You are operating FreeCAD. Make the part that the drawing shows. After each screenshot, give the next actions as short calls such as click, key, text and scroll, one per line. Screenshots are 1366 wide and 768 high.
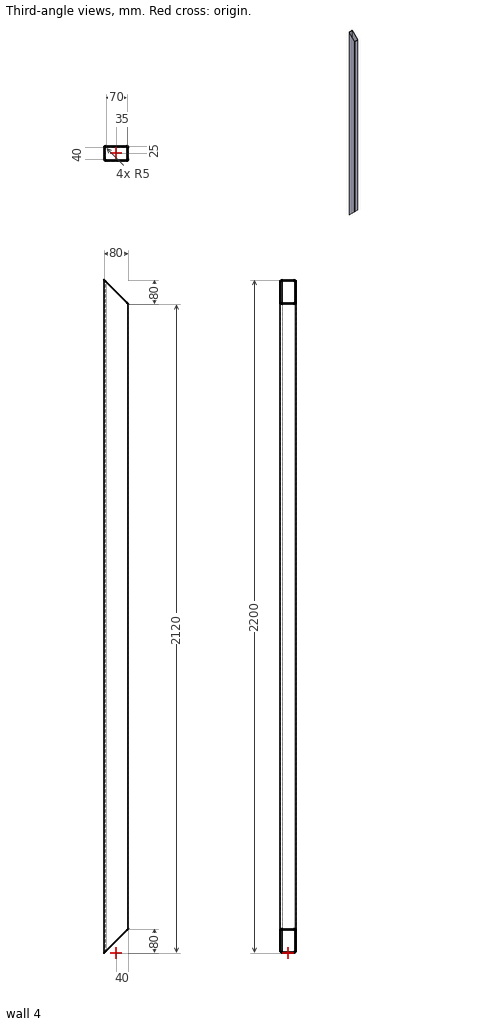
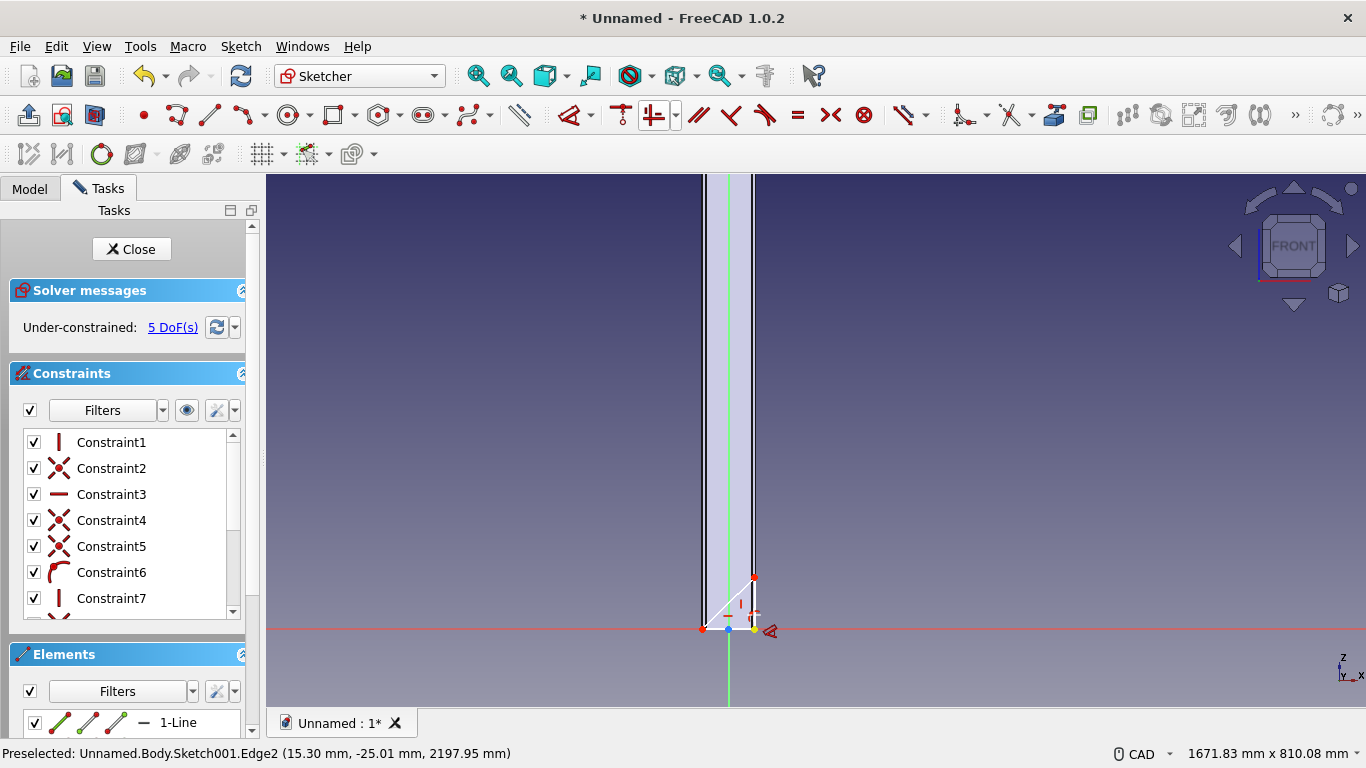
click(755, 614)
click(789, 603)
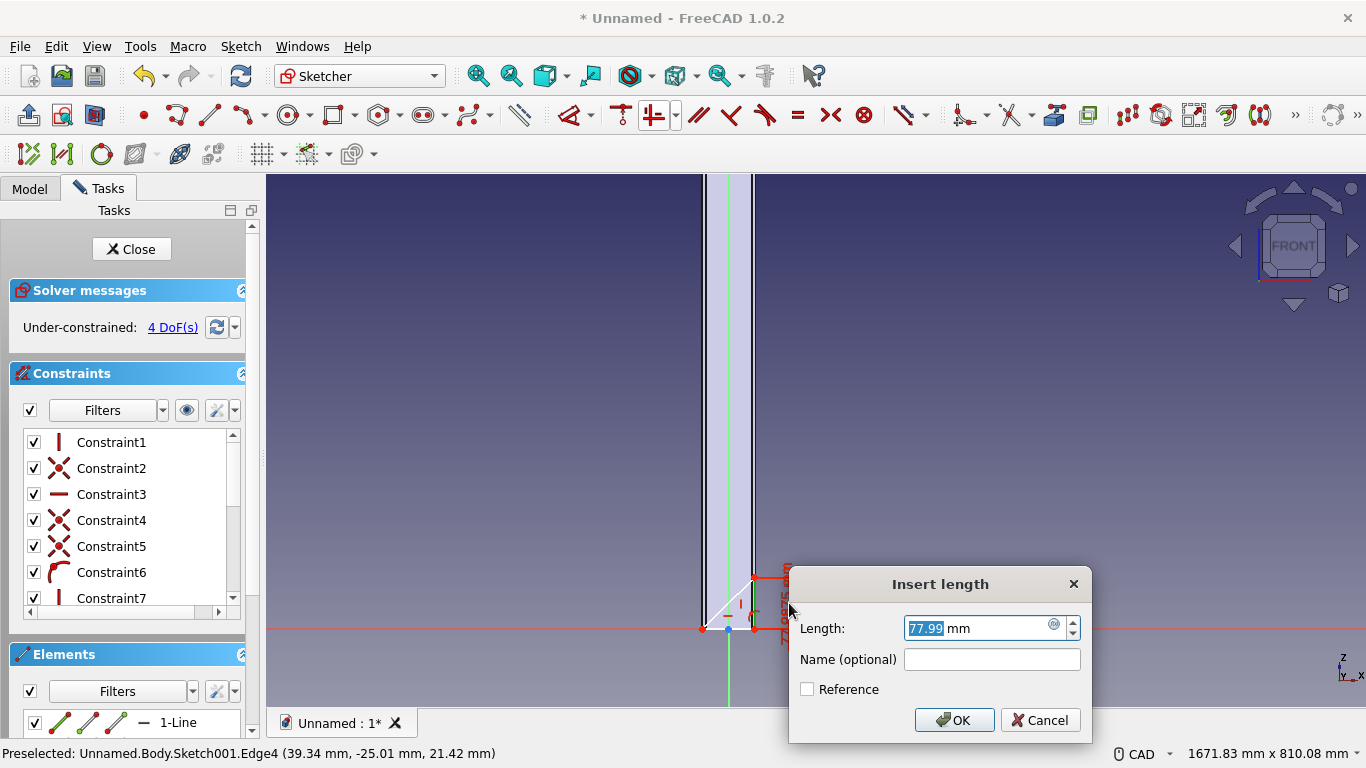
text(80)
key(Return)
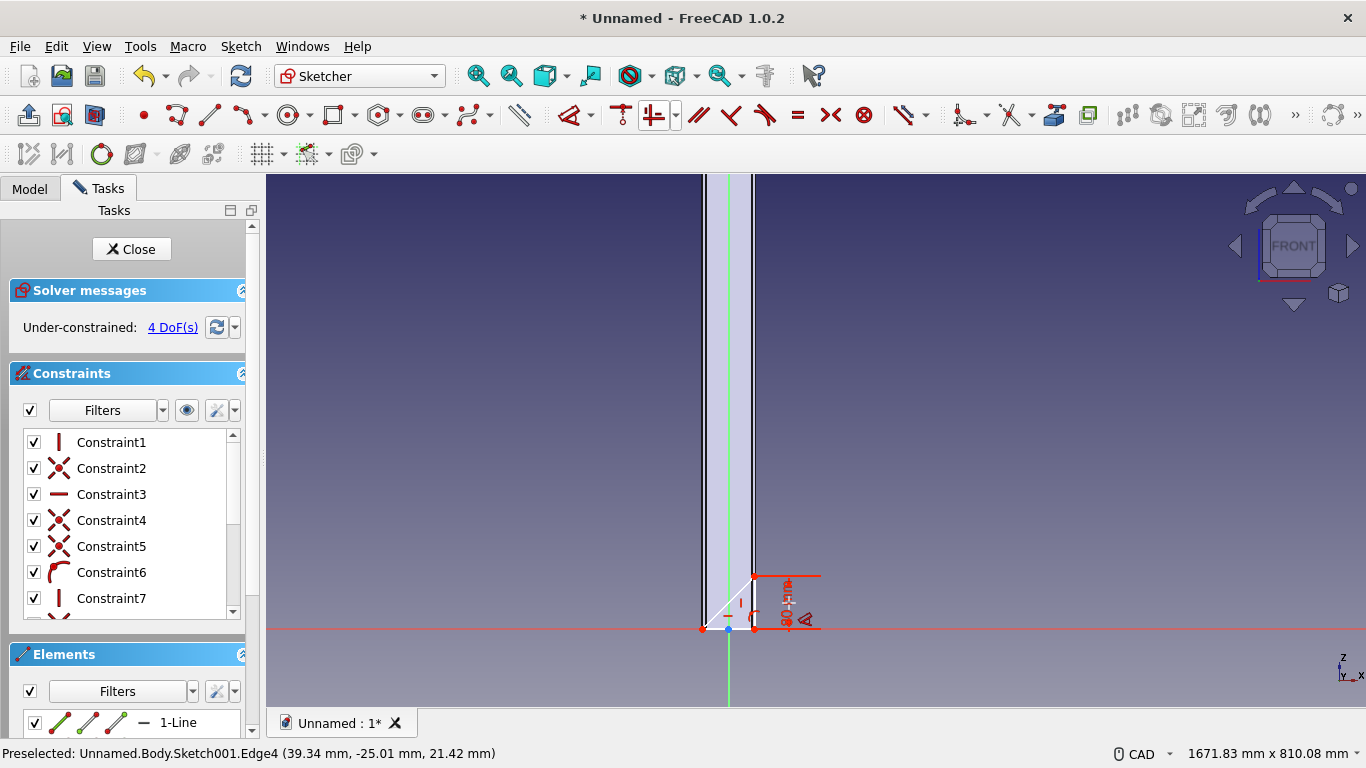
scroll(718, 629, up, 2)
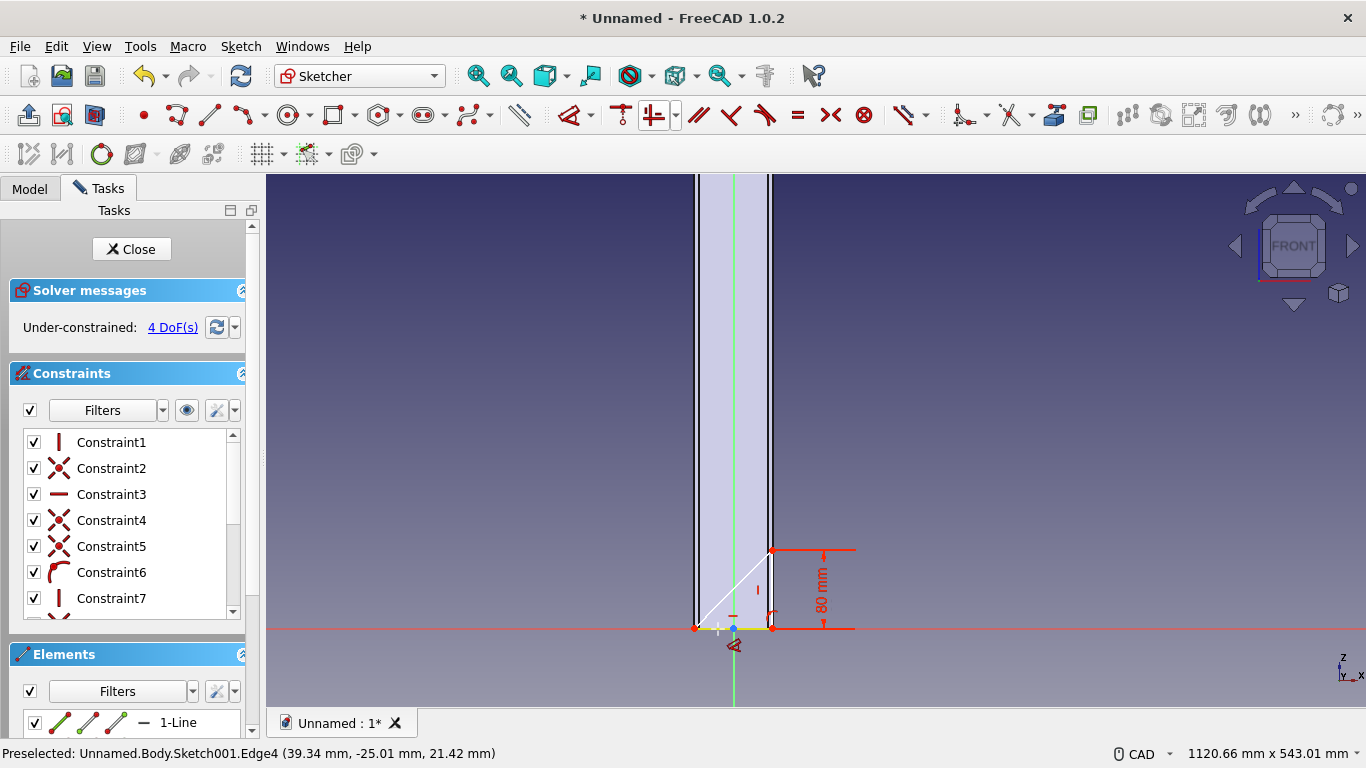
click(718, 629)
click(715, 663)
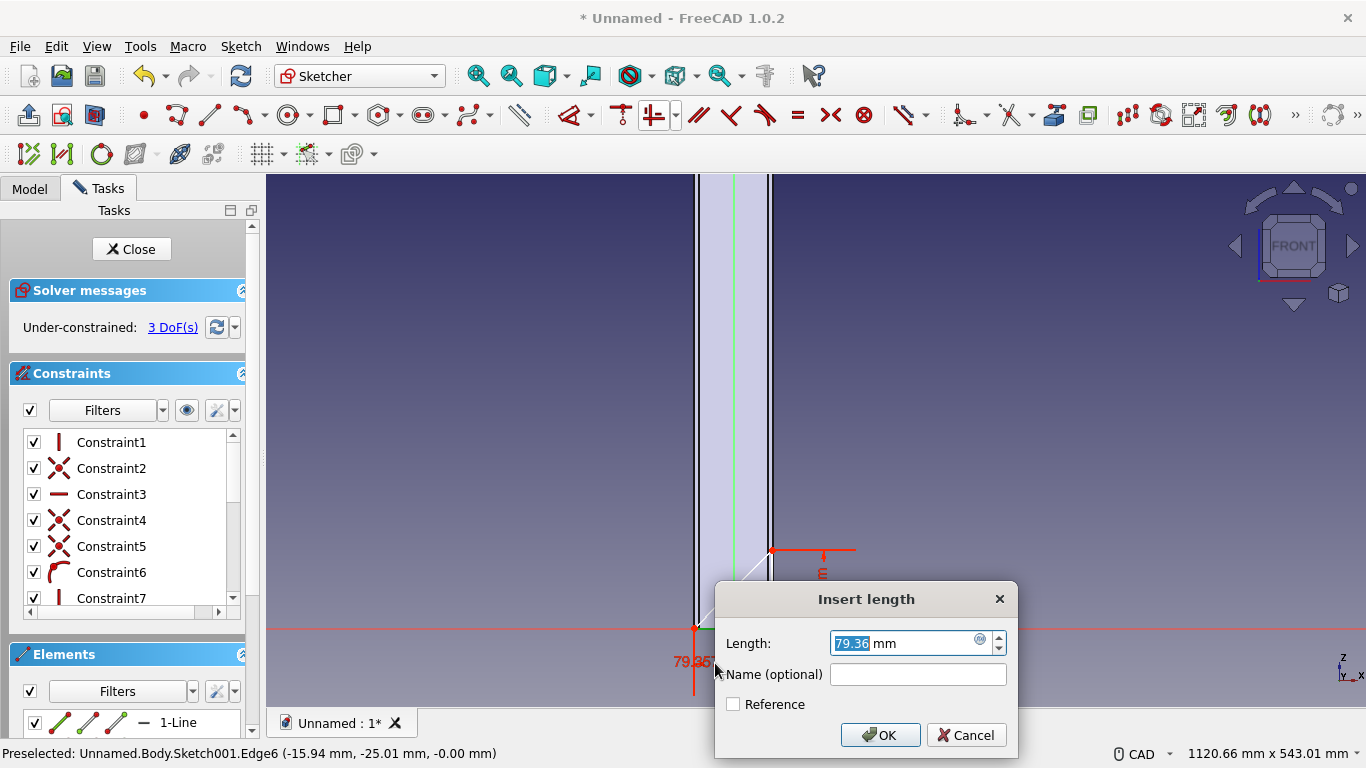
text(80)
key(Return)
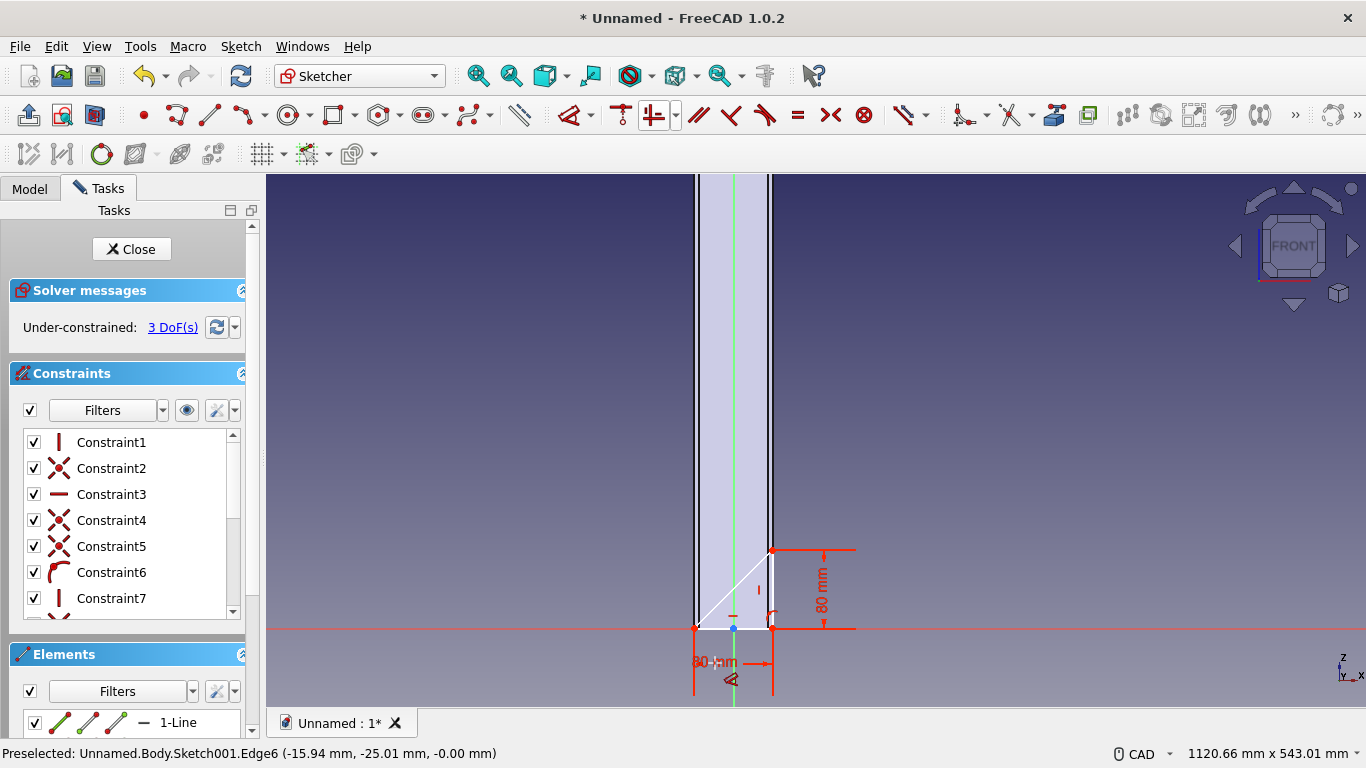
scroll(750, 617, down, 9)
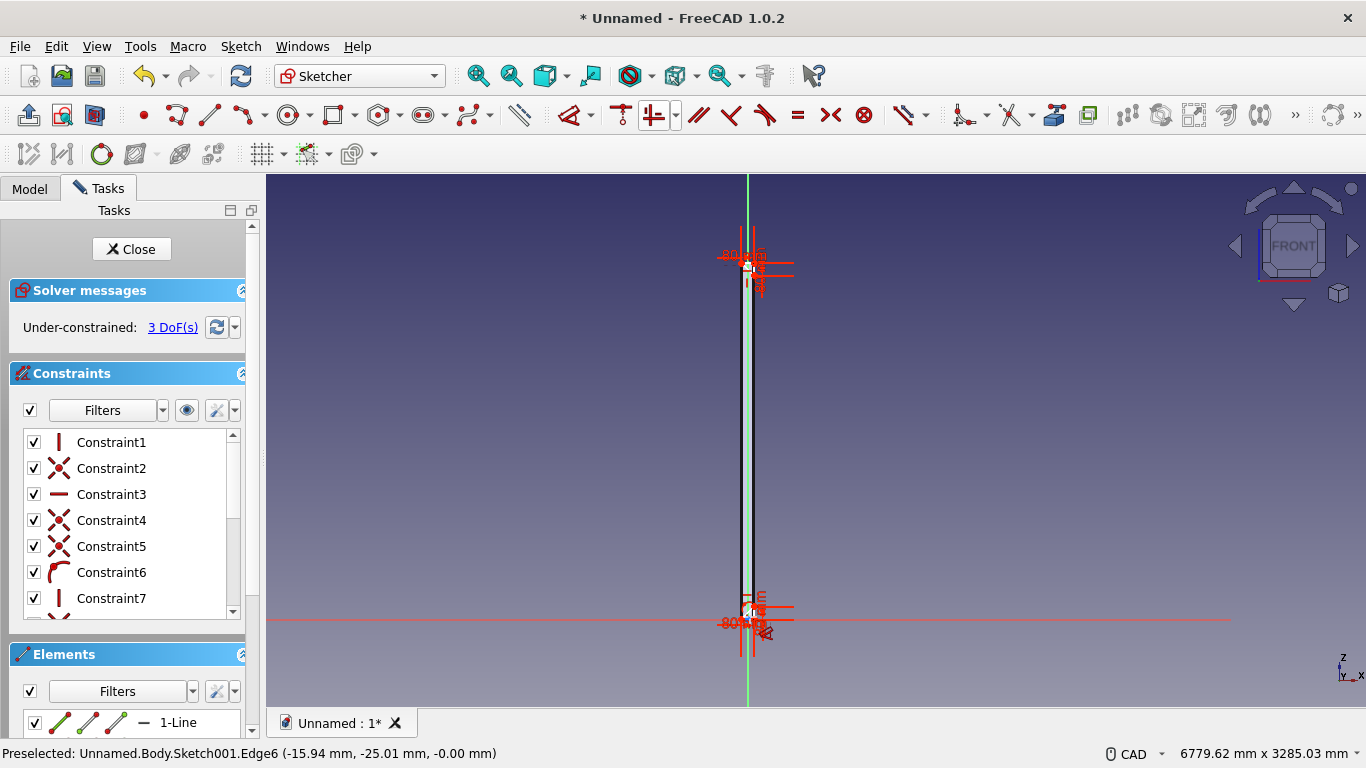
scroll(754, 276, up, 10)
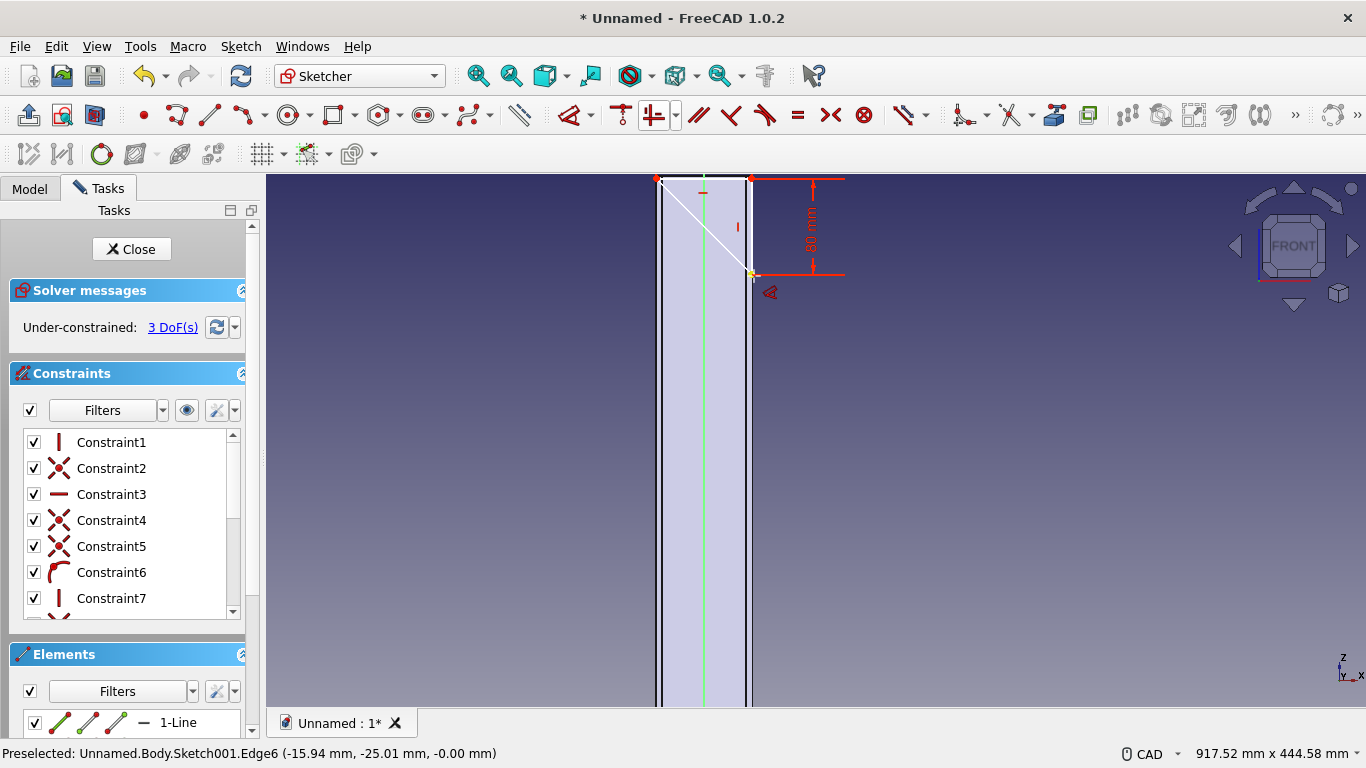
click(752, 275)
click(728, 217)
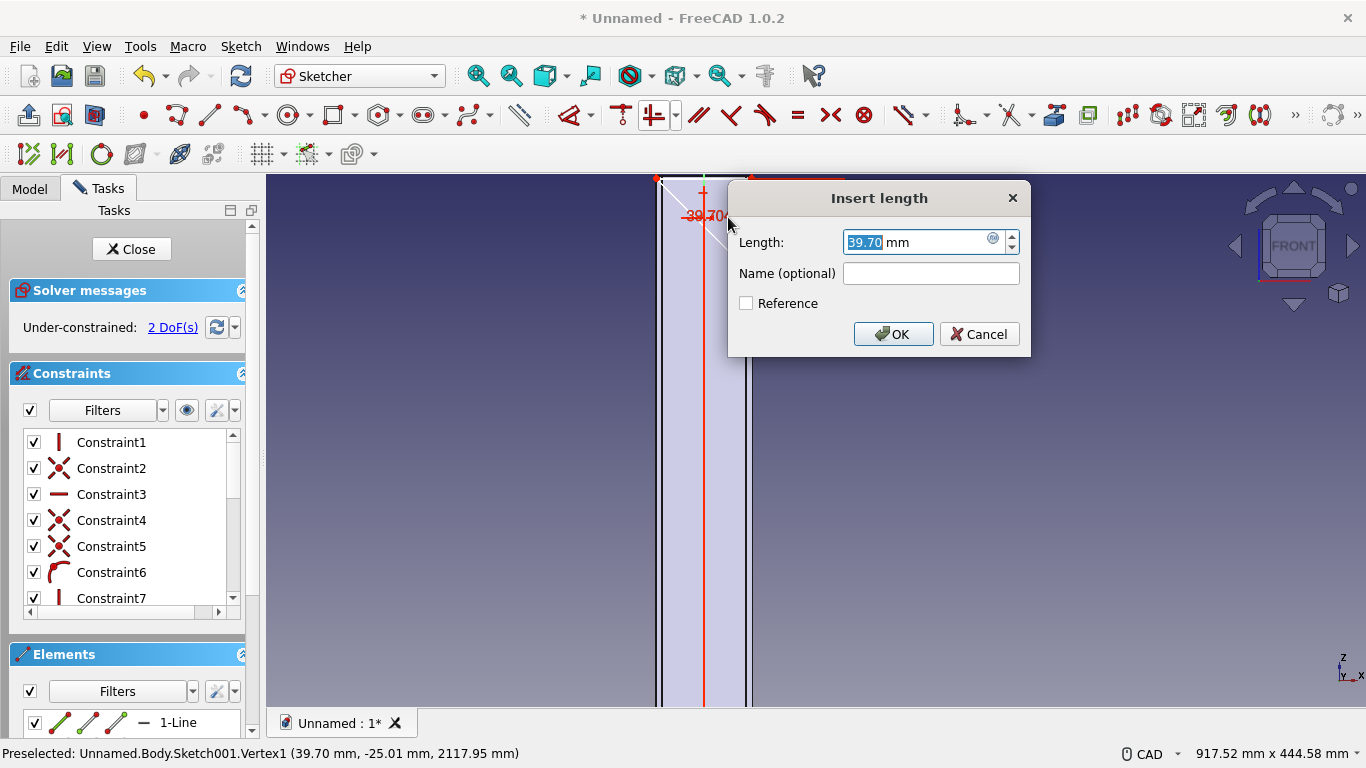
text(40)
key(Return)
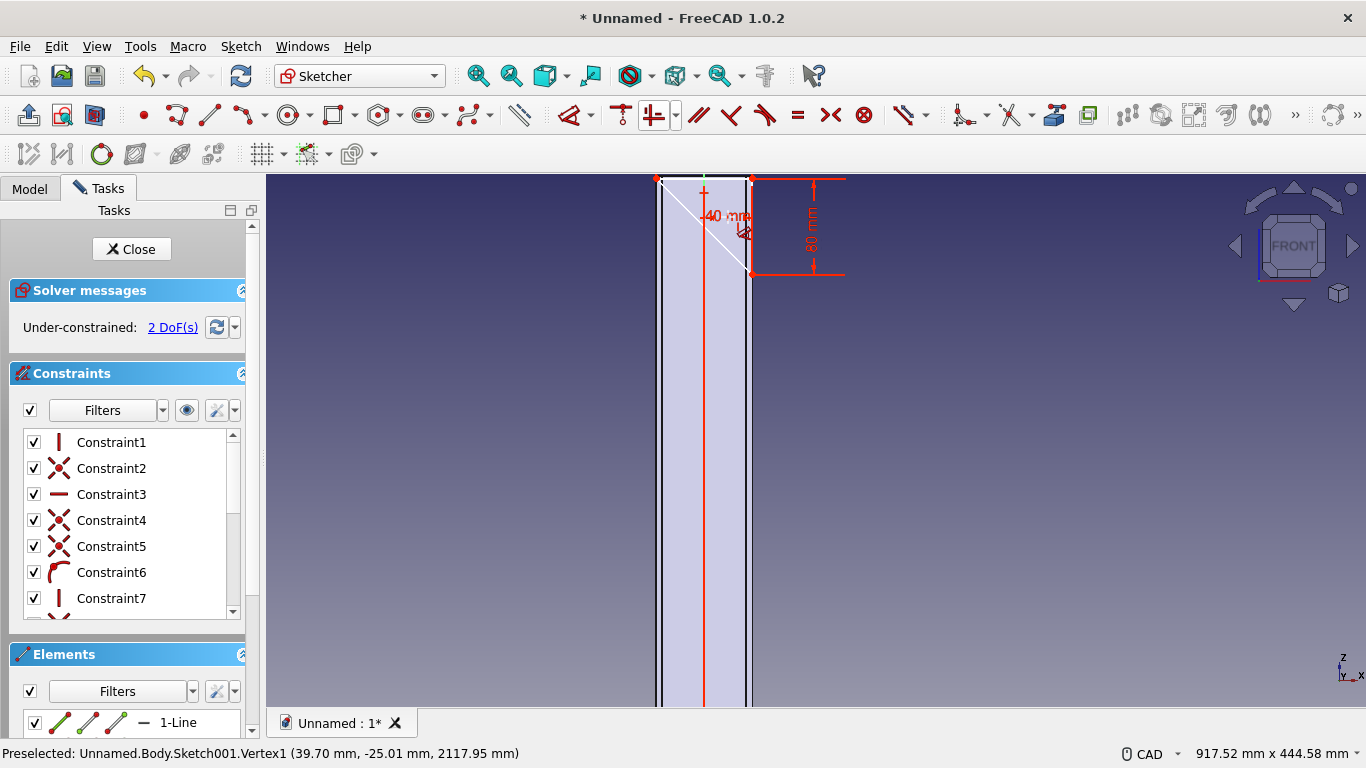
scroll(754, 275, down, 10)